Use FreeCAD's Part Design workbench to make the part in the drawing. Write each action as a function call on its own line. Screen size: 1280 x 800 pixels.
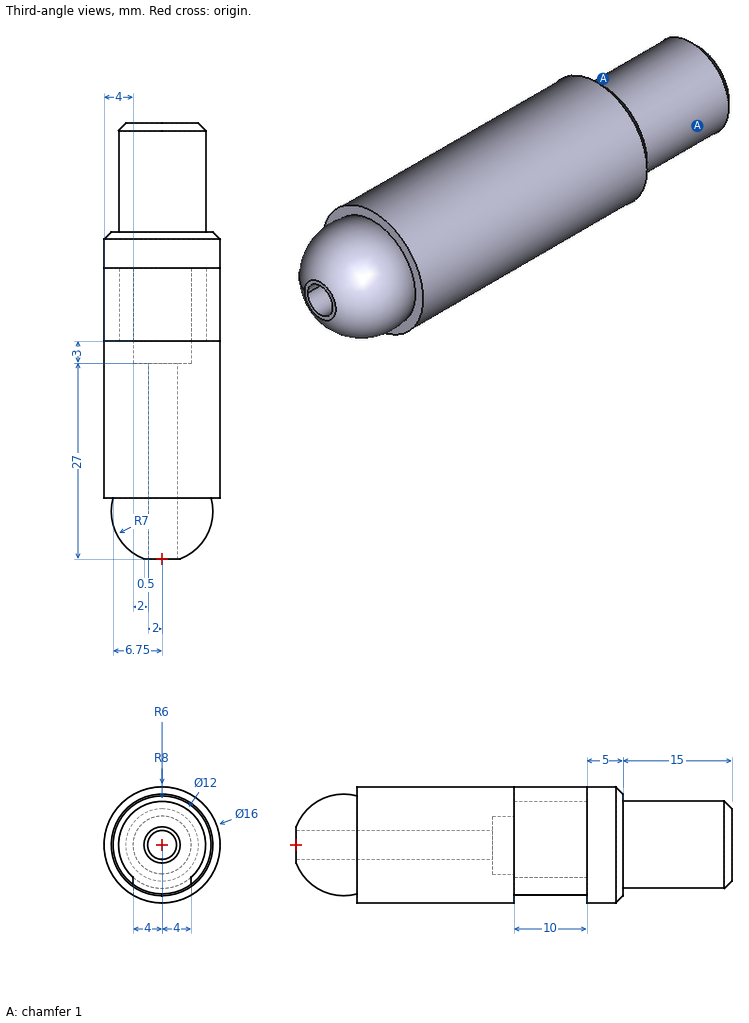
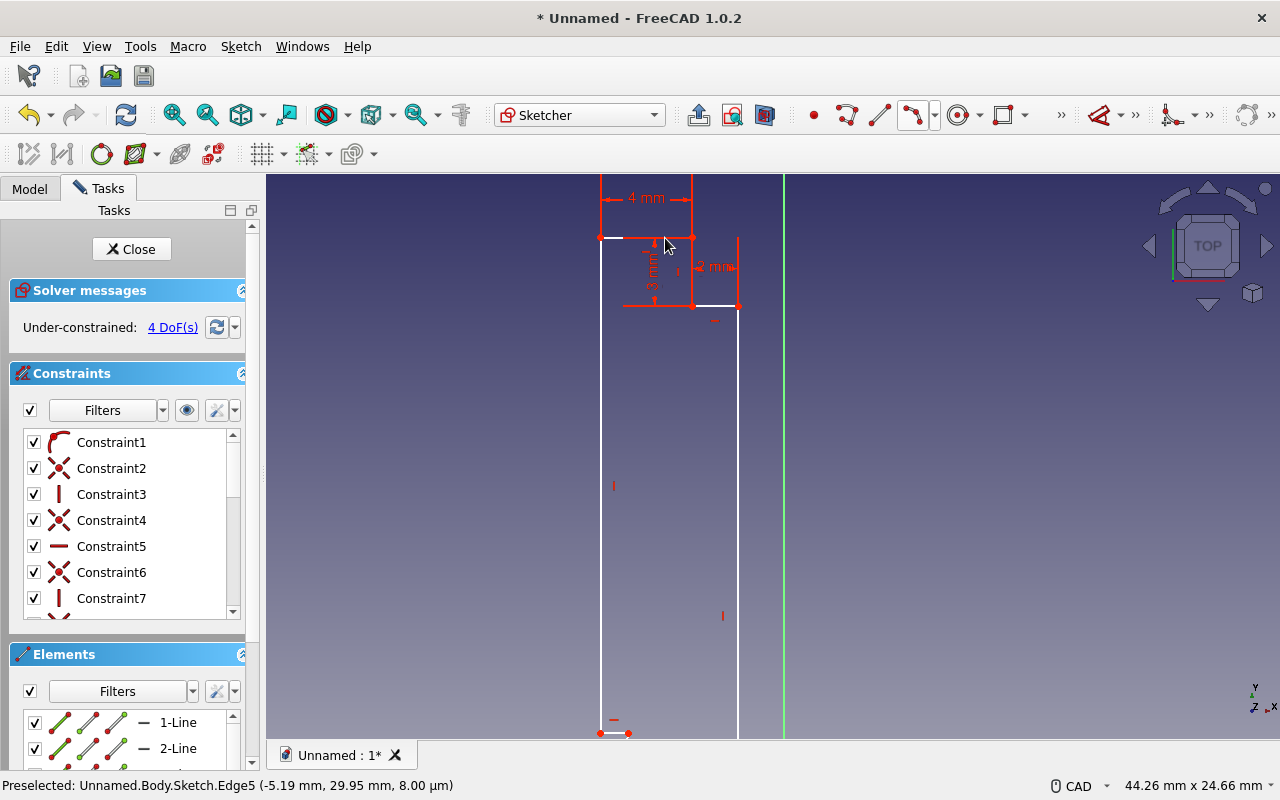
click(738, 492)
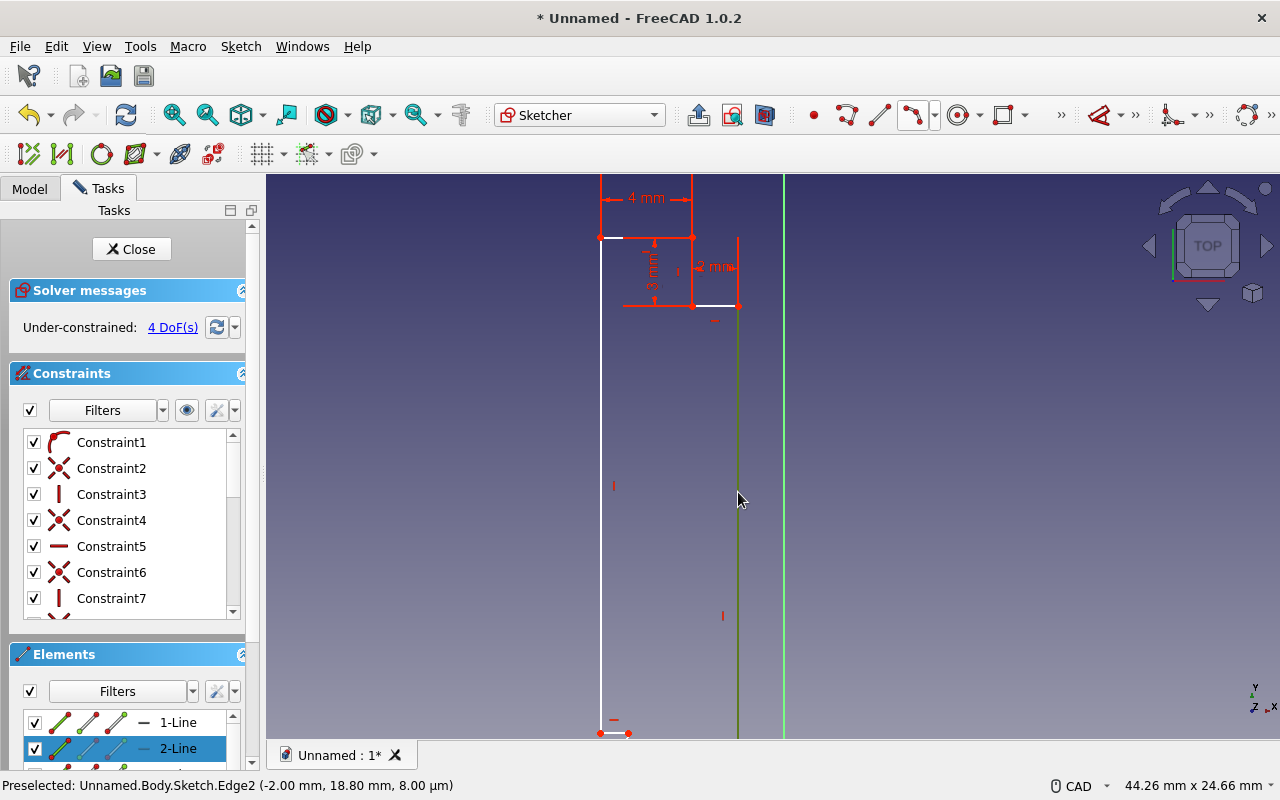
key(i)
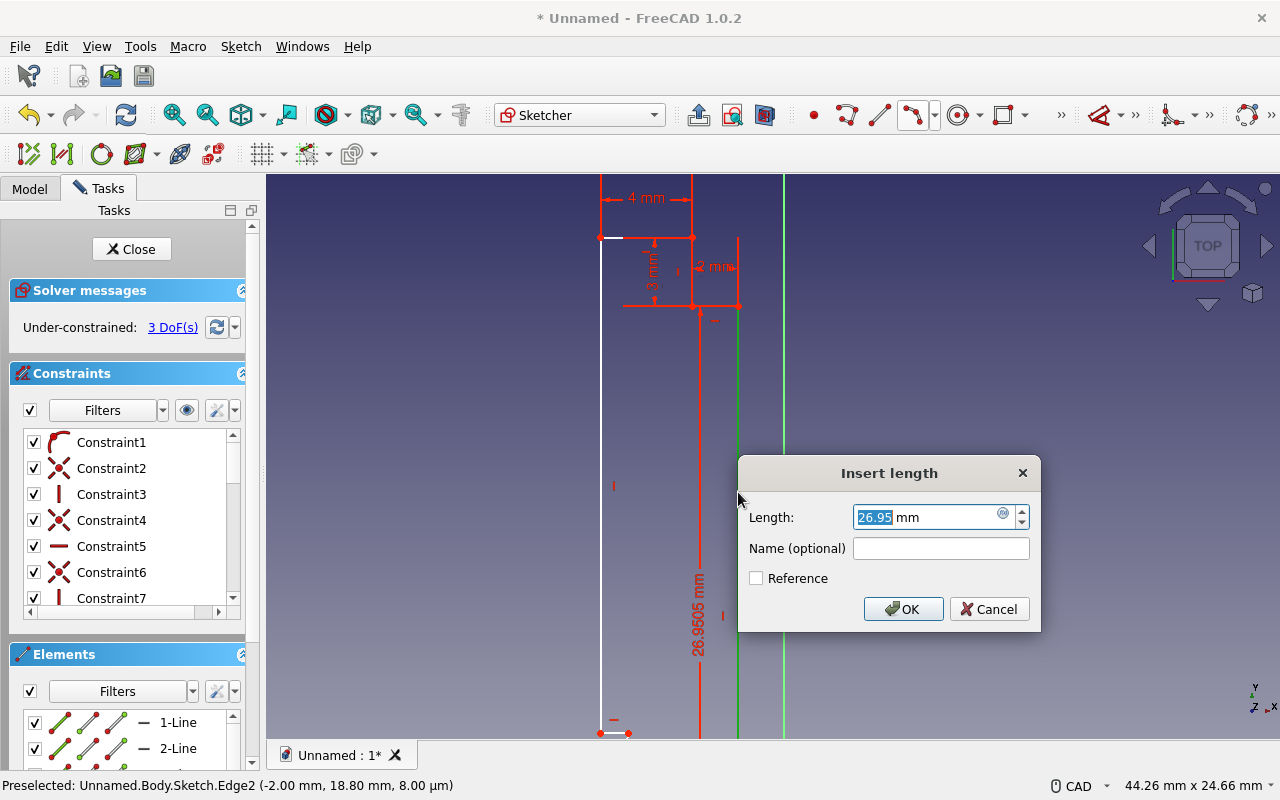
text(27)
key(Return)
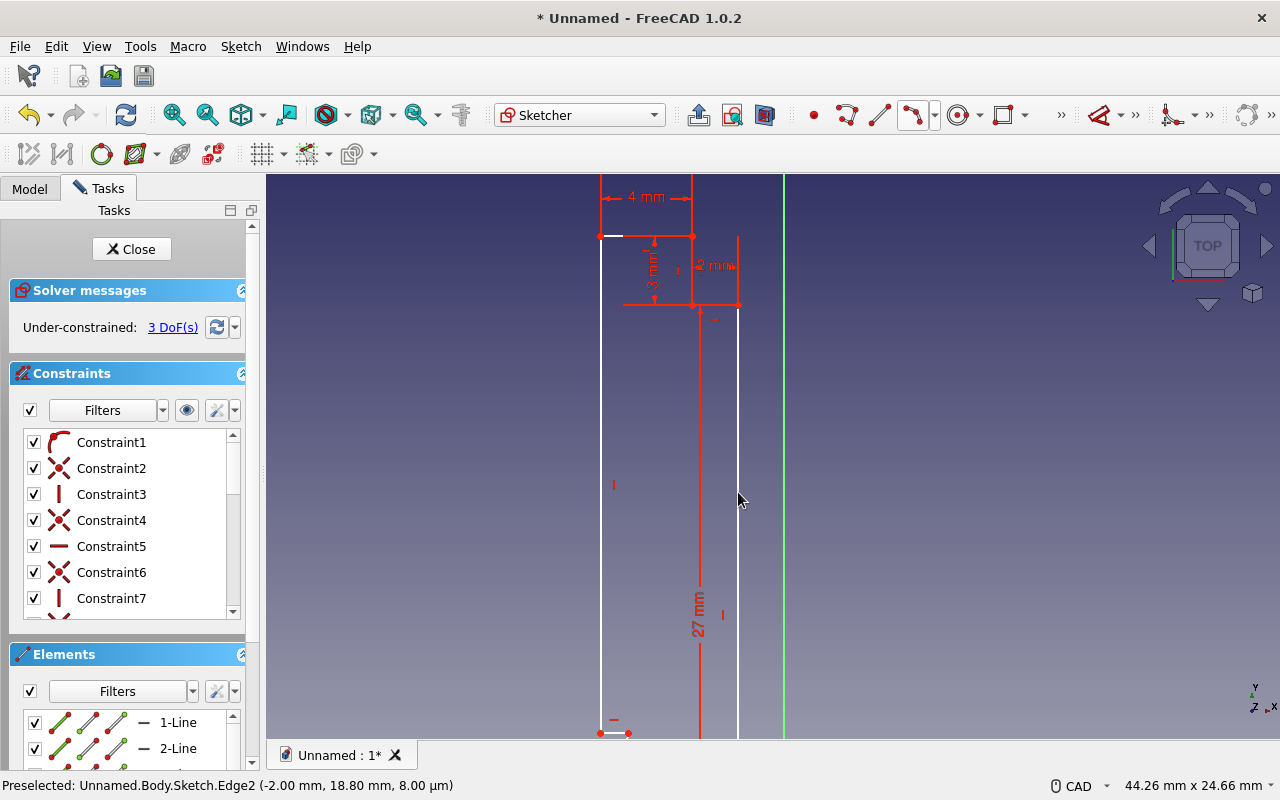
scroll(719, 306, down, 3)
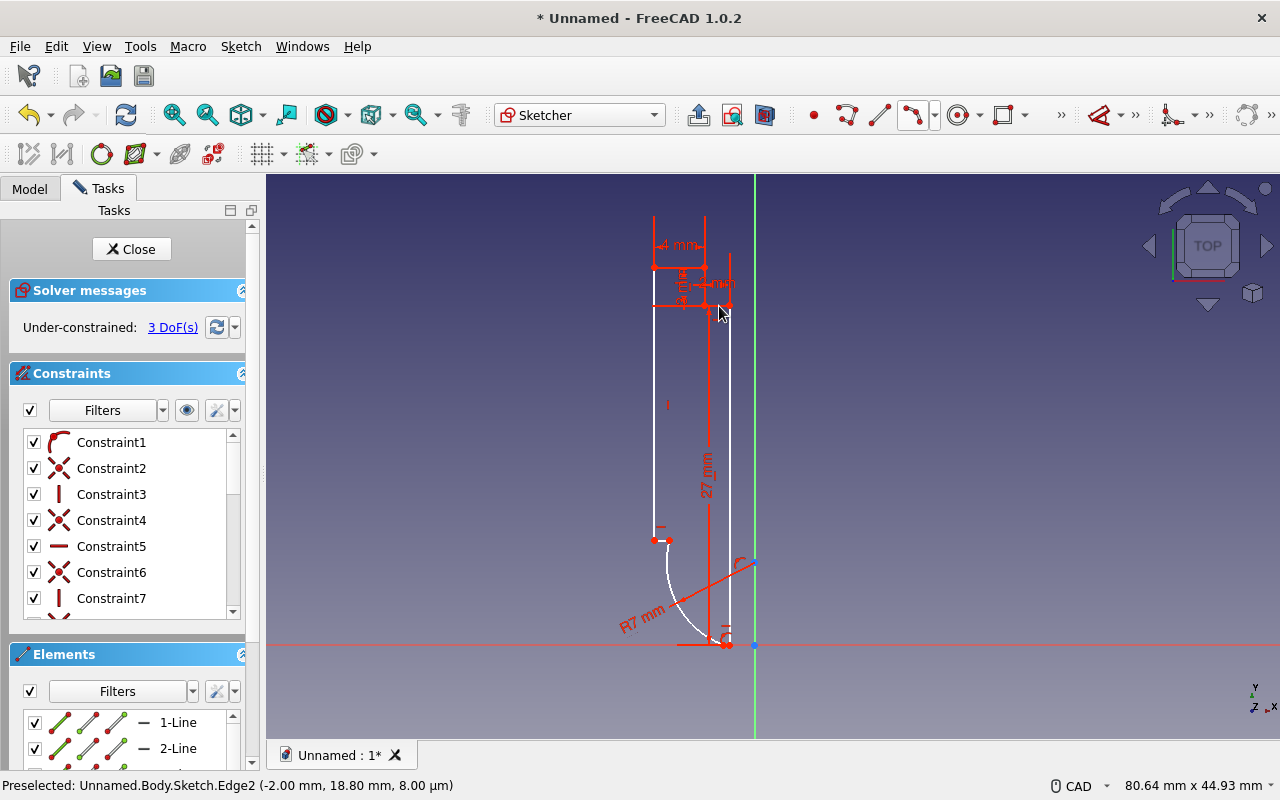
scroll(730, 645, up, 4)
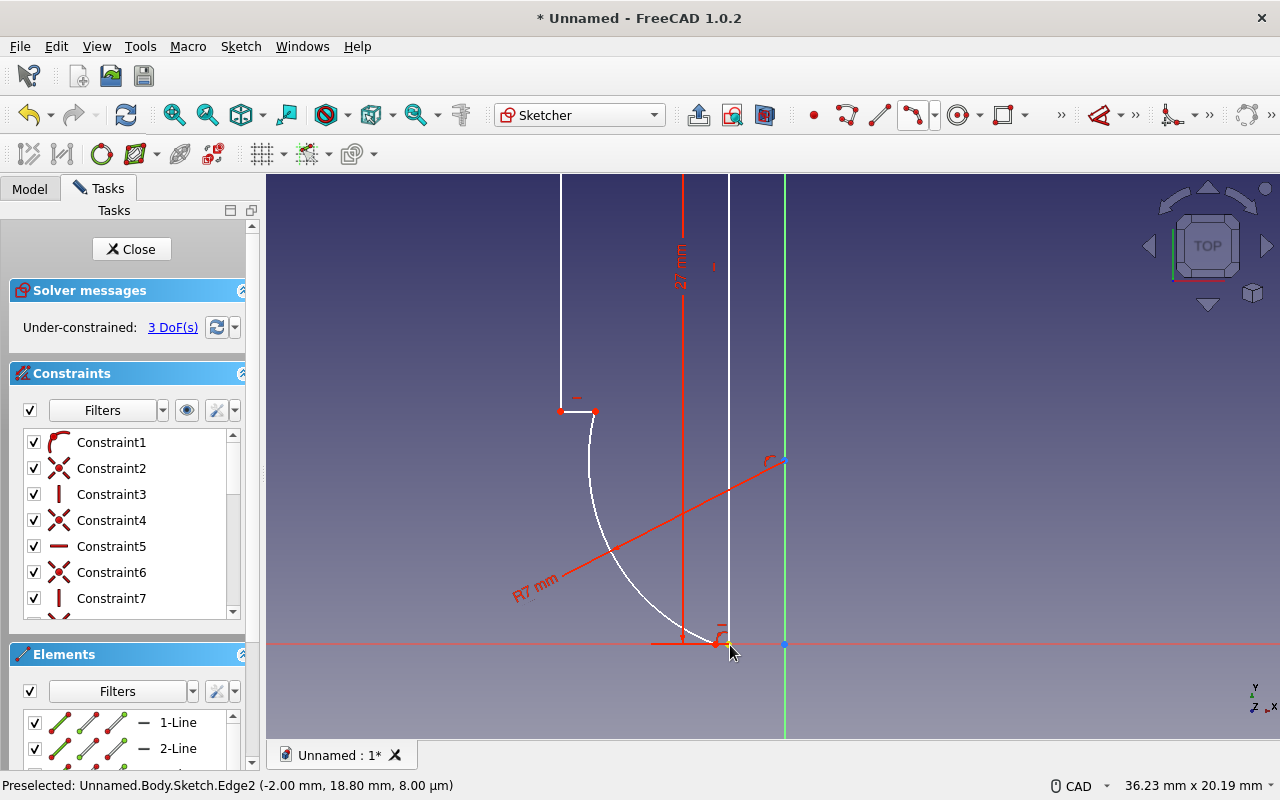
click(729, 644)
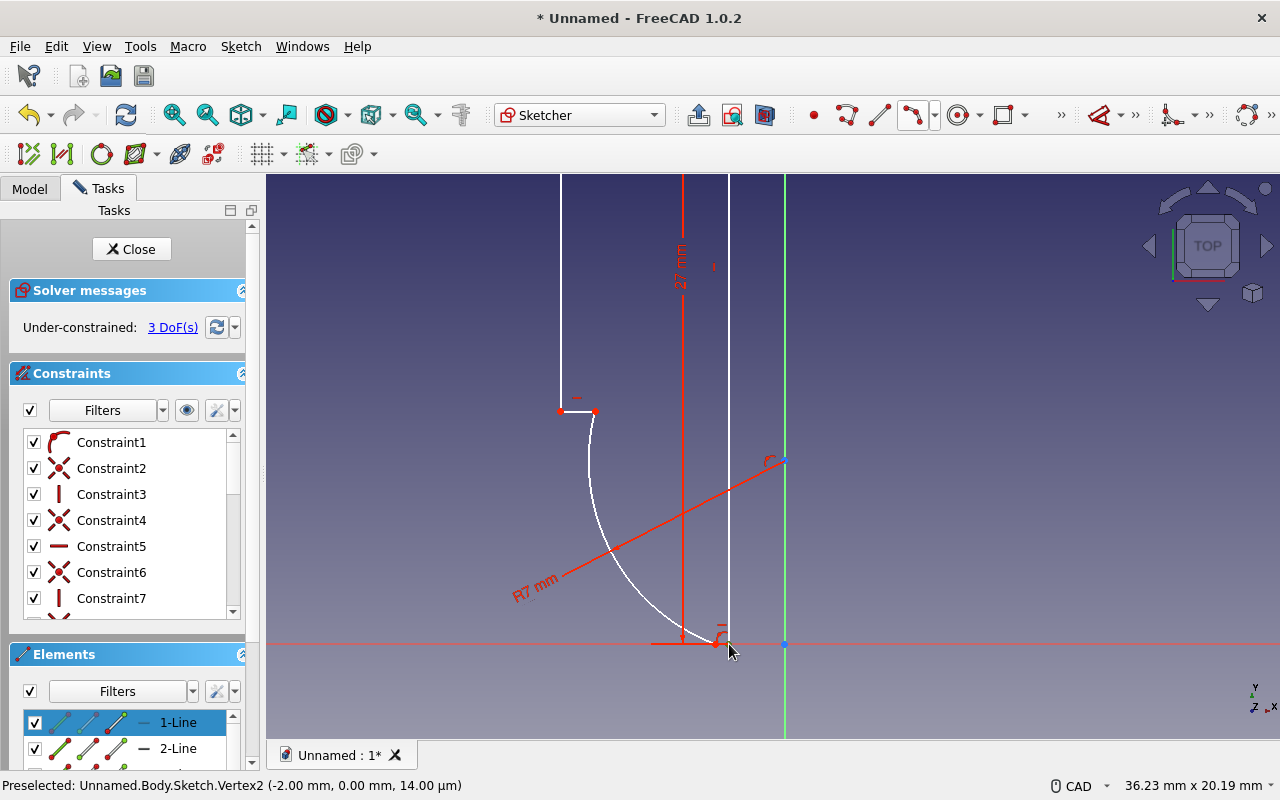
click(1120, 116)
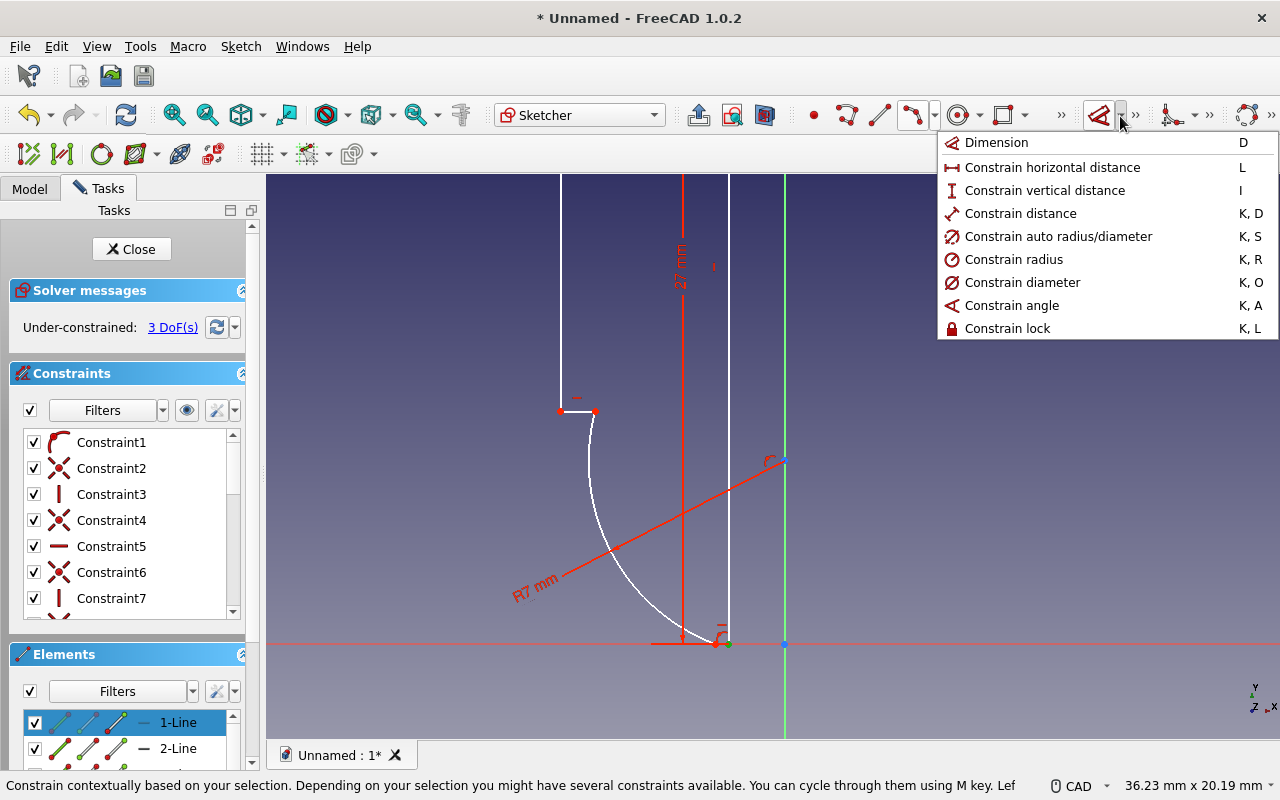
click(1108, 168)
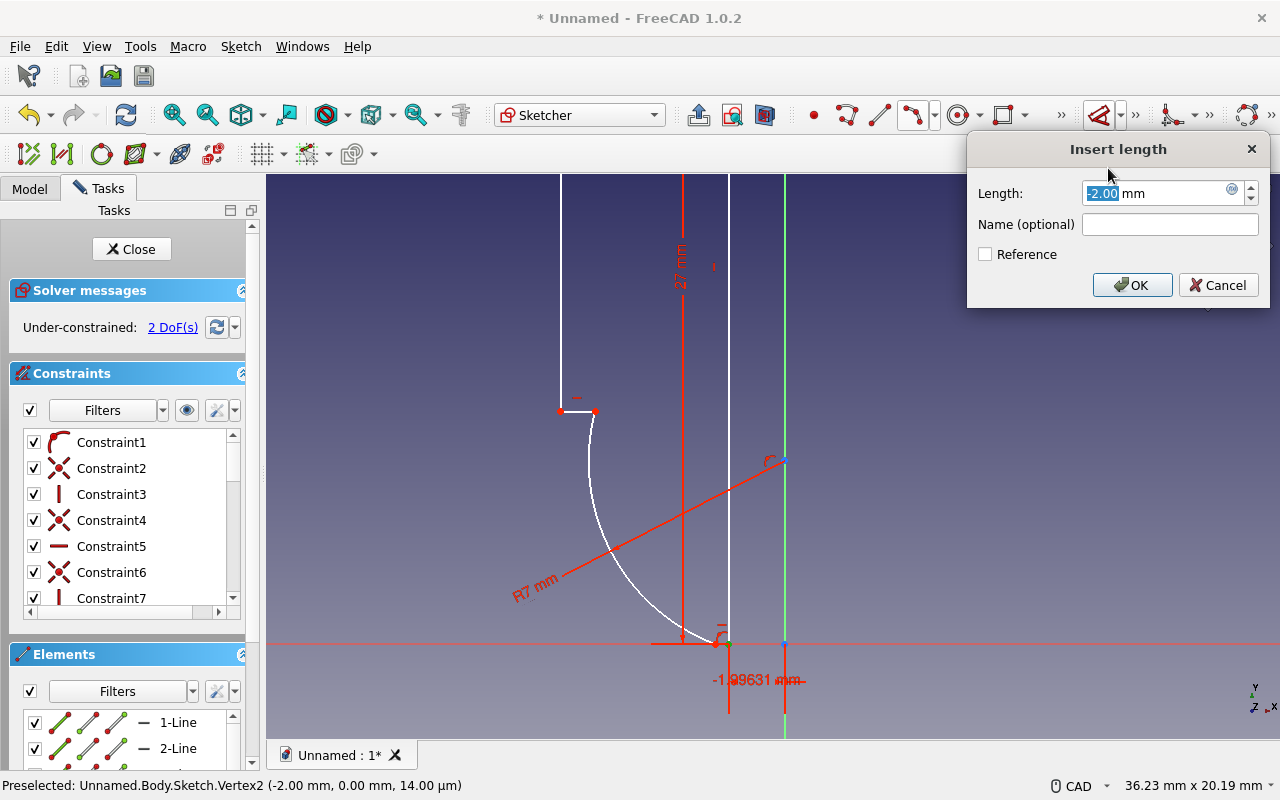
text(-2)
key(Return)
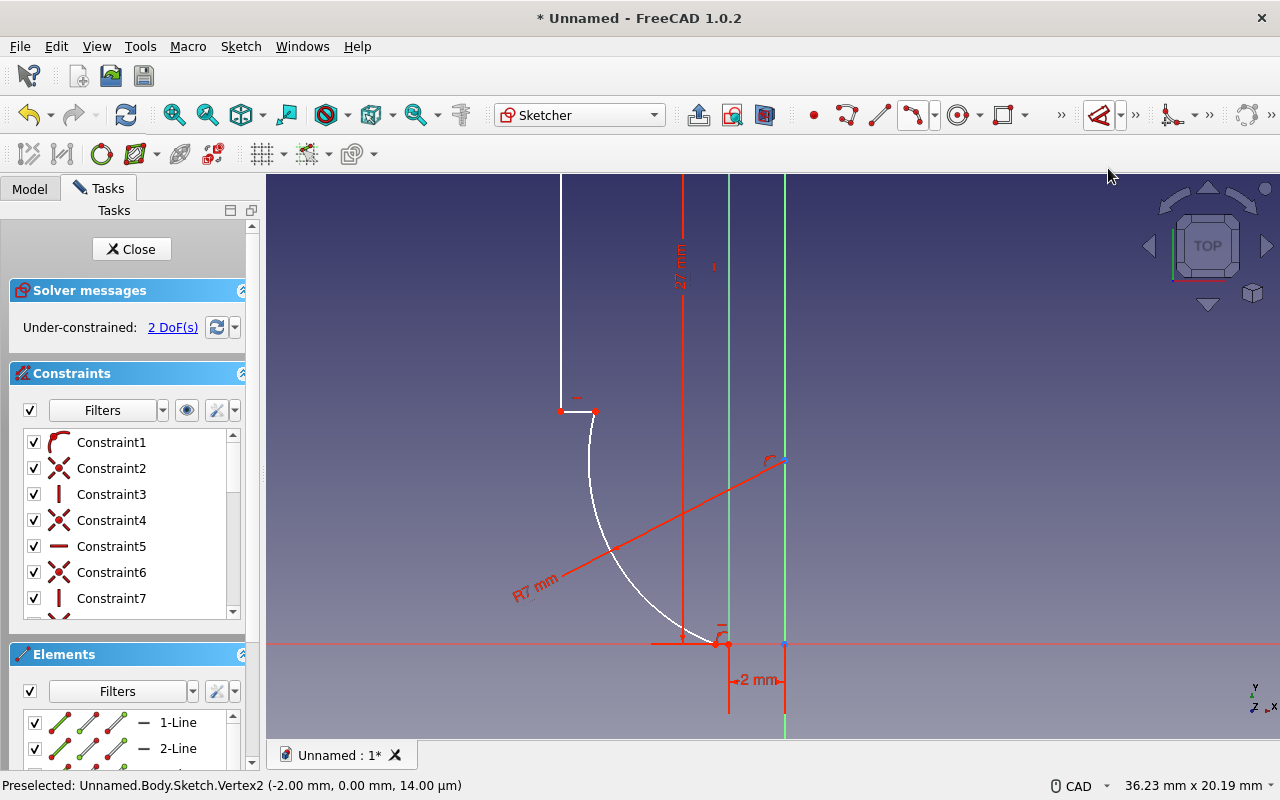
scroll(722, 644, up, 6)